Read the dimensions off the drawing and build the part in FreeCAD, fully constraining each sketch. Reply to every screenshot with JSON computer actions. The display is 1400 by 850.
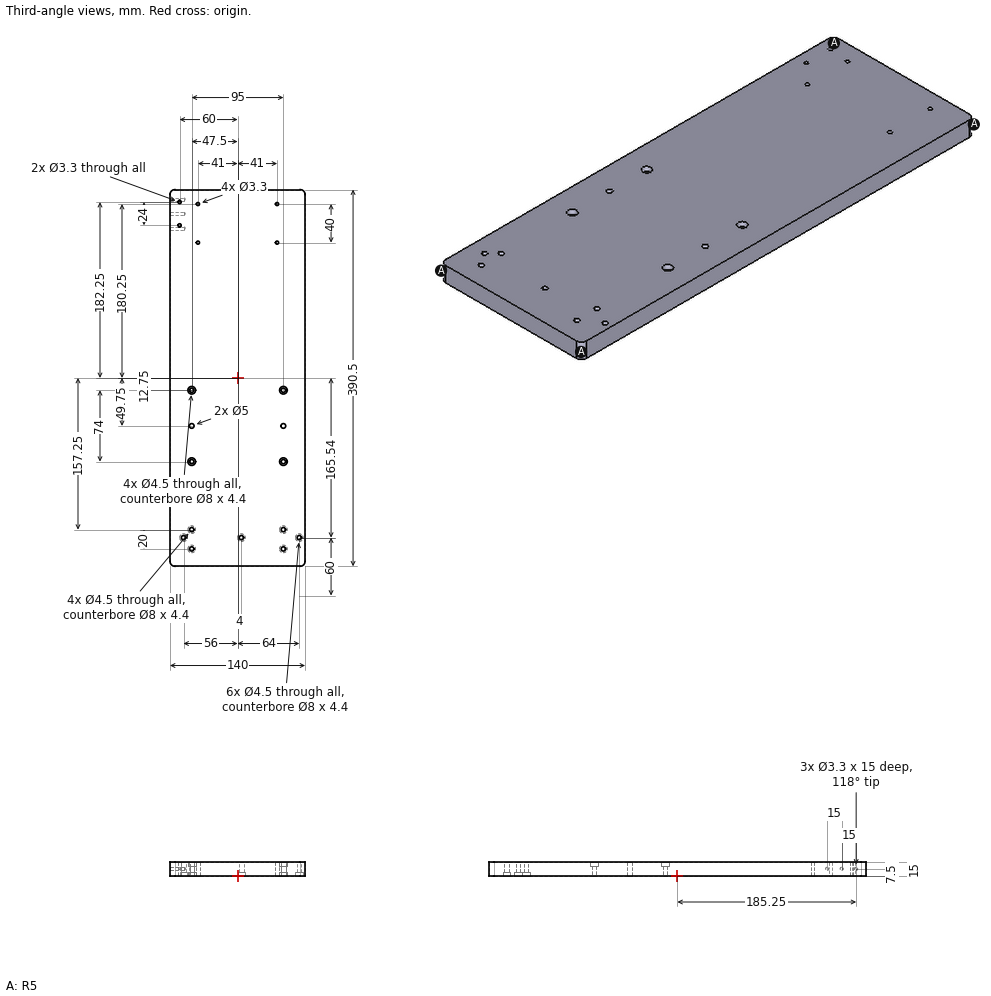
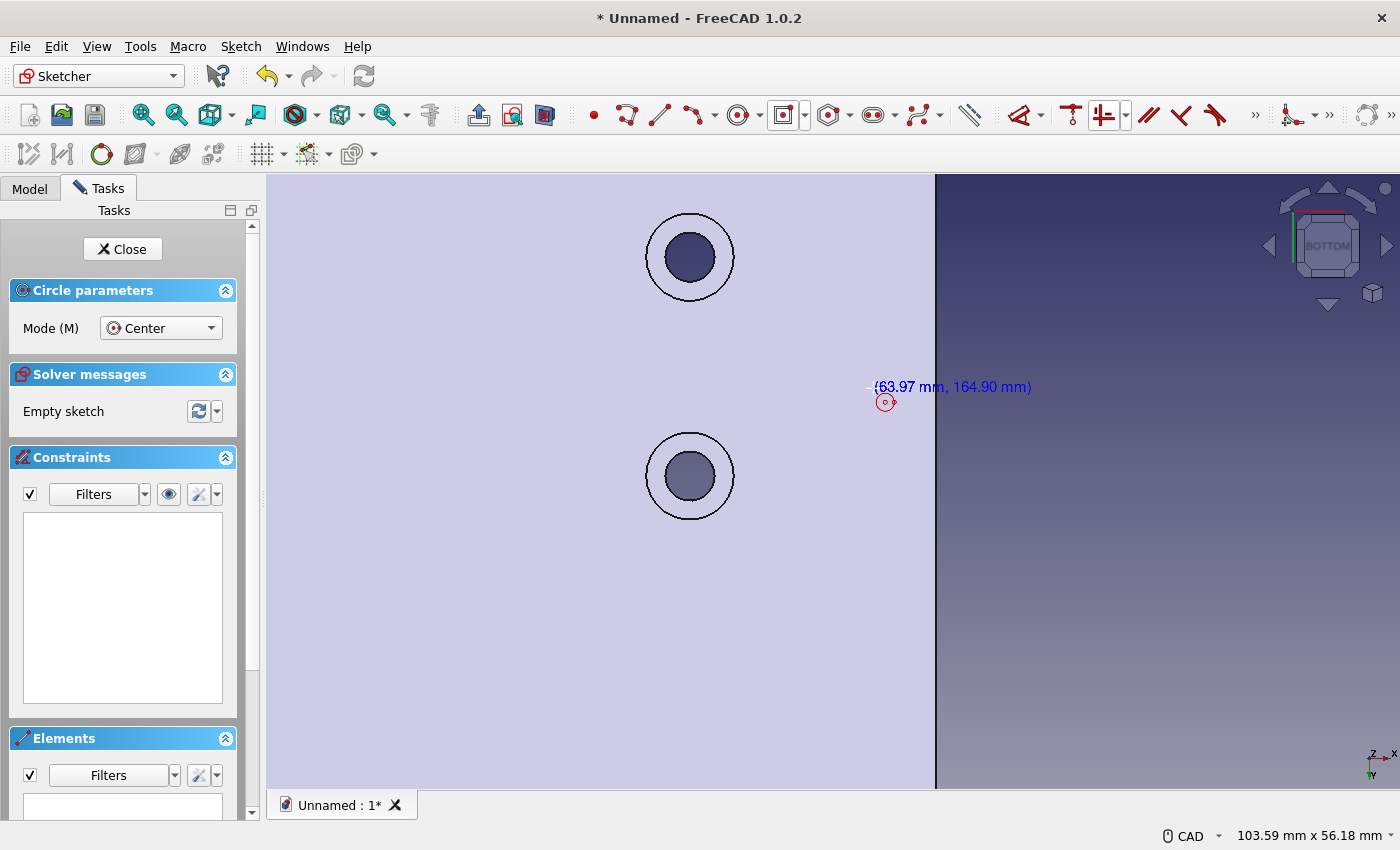
{"action": "scroll", "coordinate": [874, 389], "scroll_direction": "down", "scroll_amount": 9}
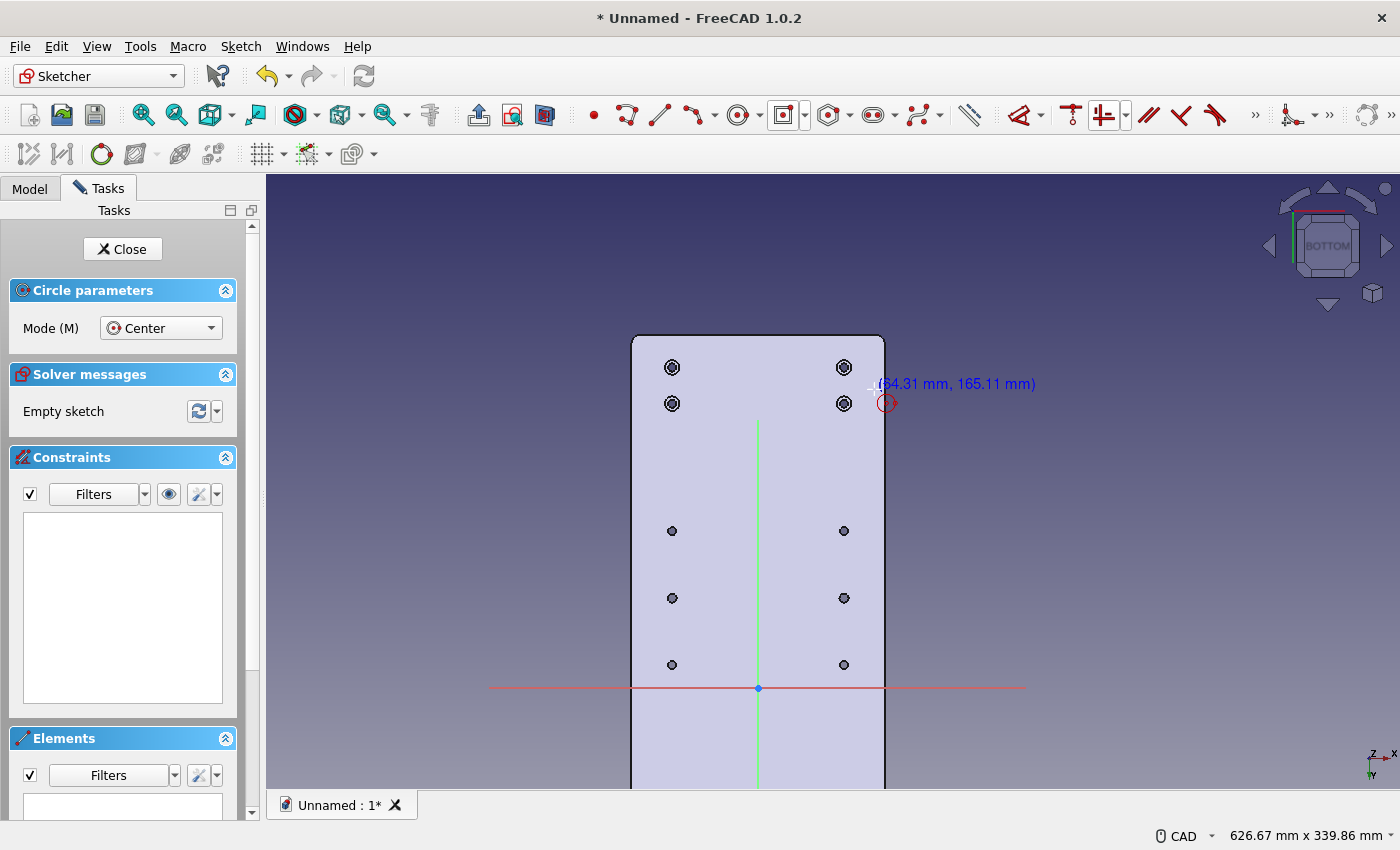
{"action": "left_click", "coordinate": [874, 389]}
{"action": "mouse_move", "coordinate": [877, 386]}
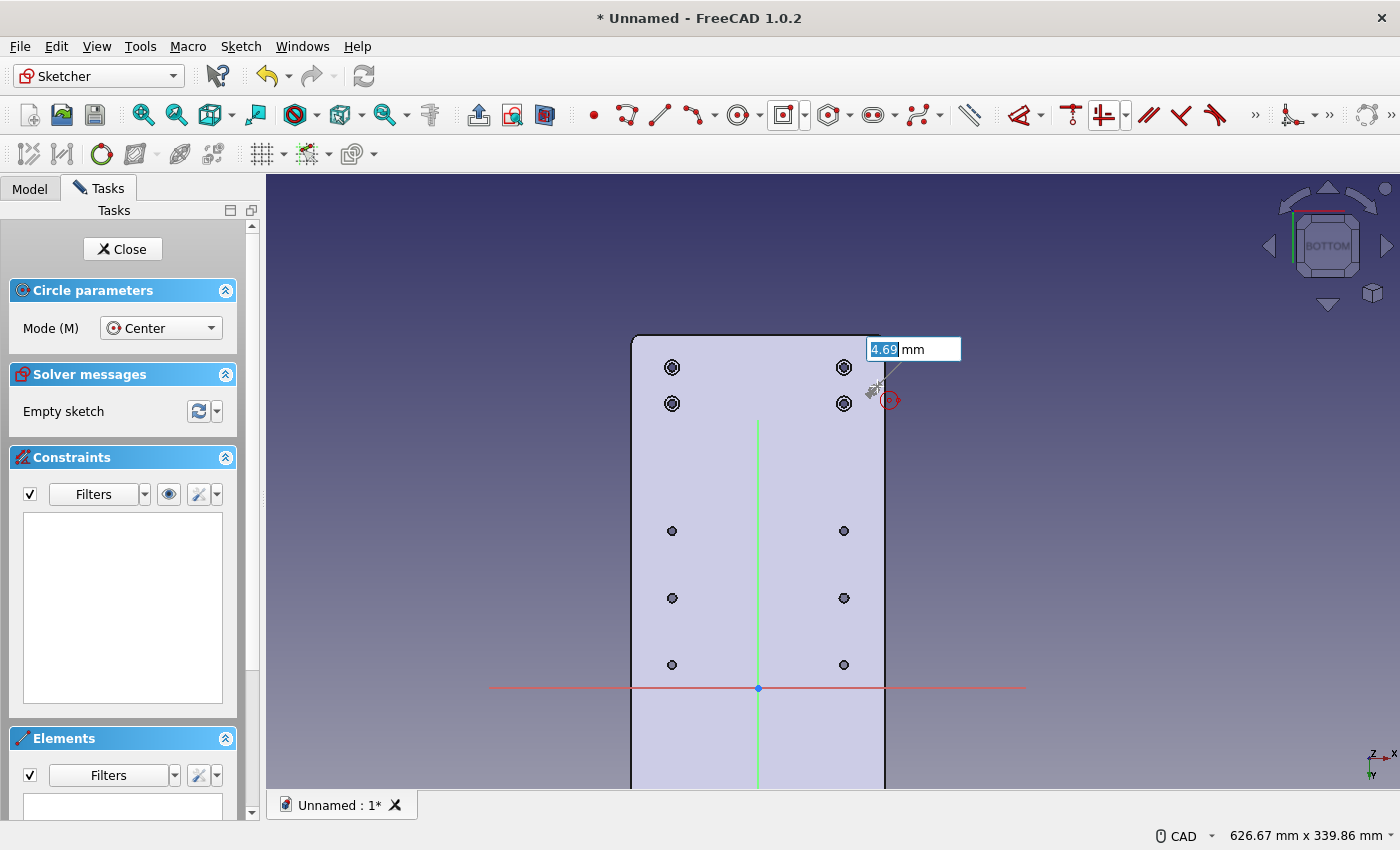
{"action": "type", "text": "4.5"}
{"action": "key", "text": "Return"}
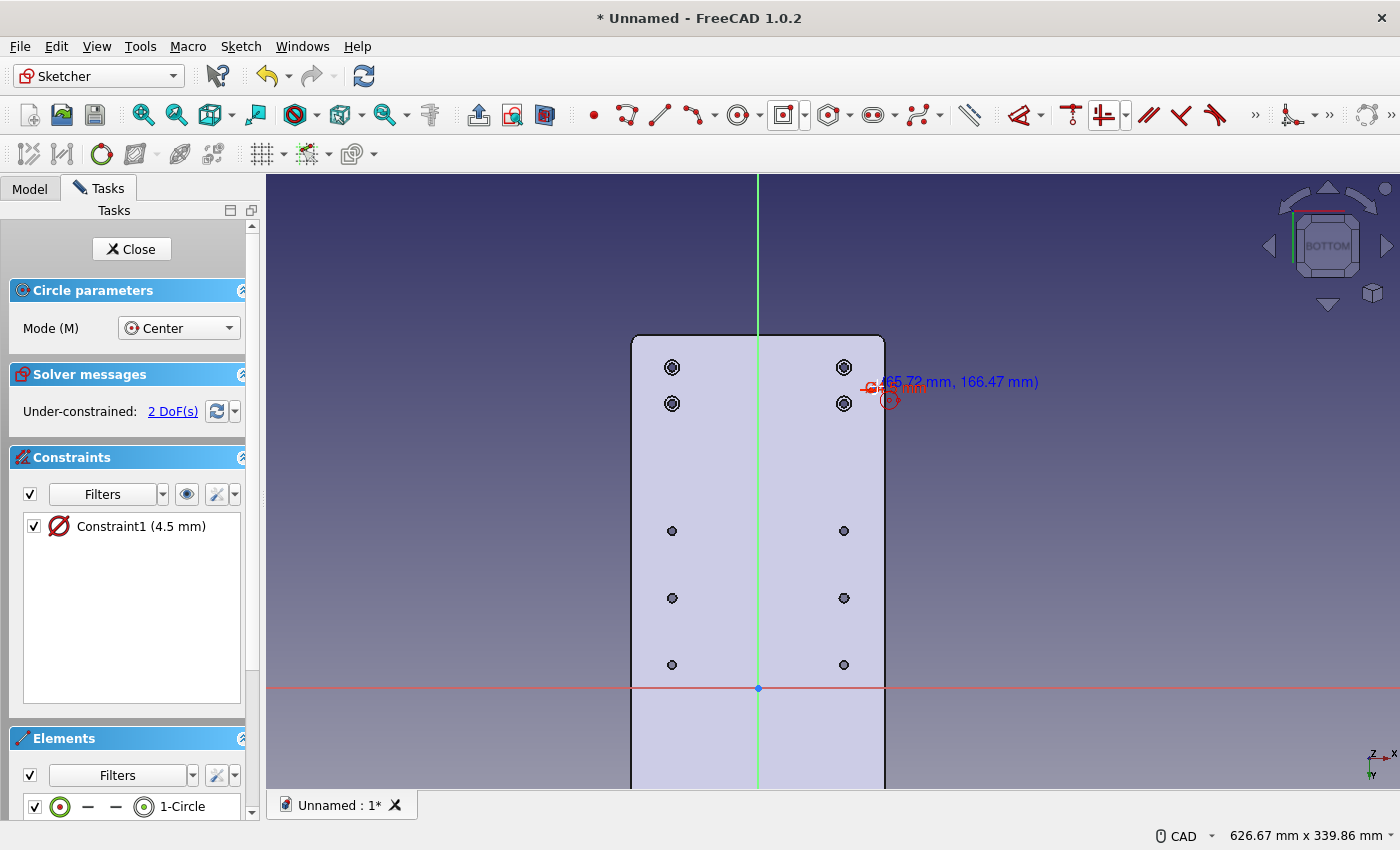
{"action": "scroll", "coordinate": [765, 389], "scroll_direction": "up", "scroll_amount": 9}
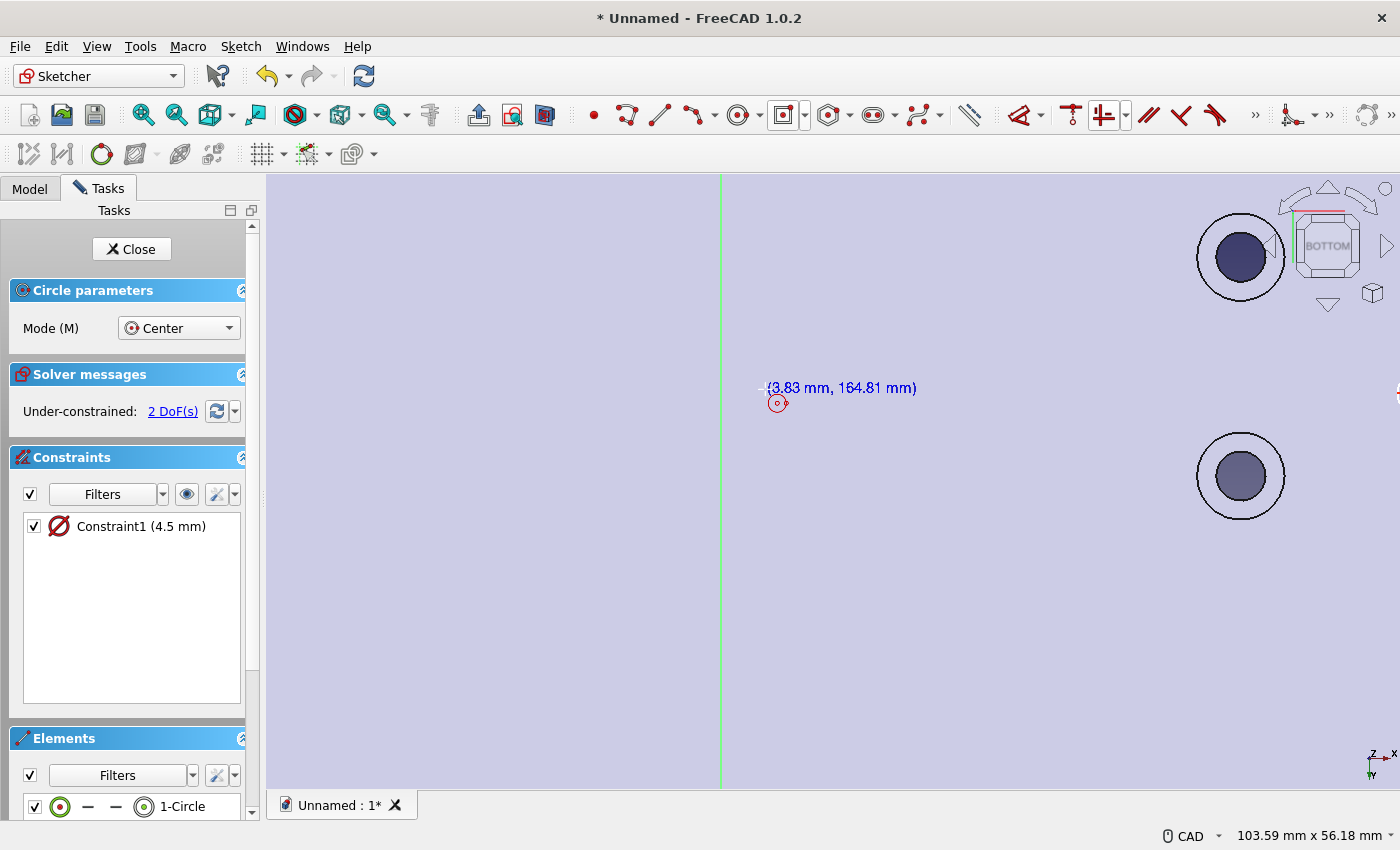
{"action": "left_click", "coordinate": [765, 385]}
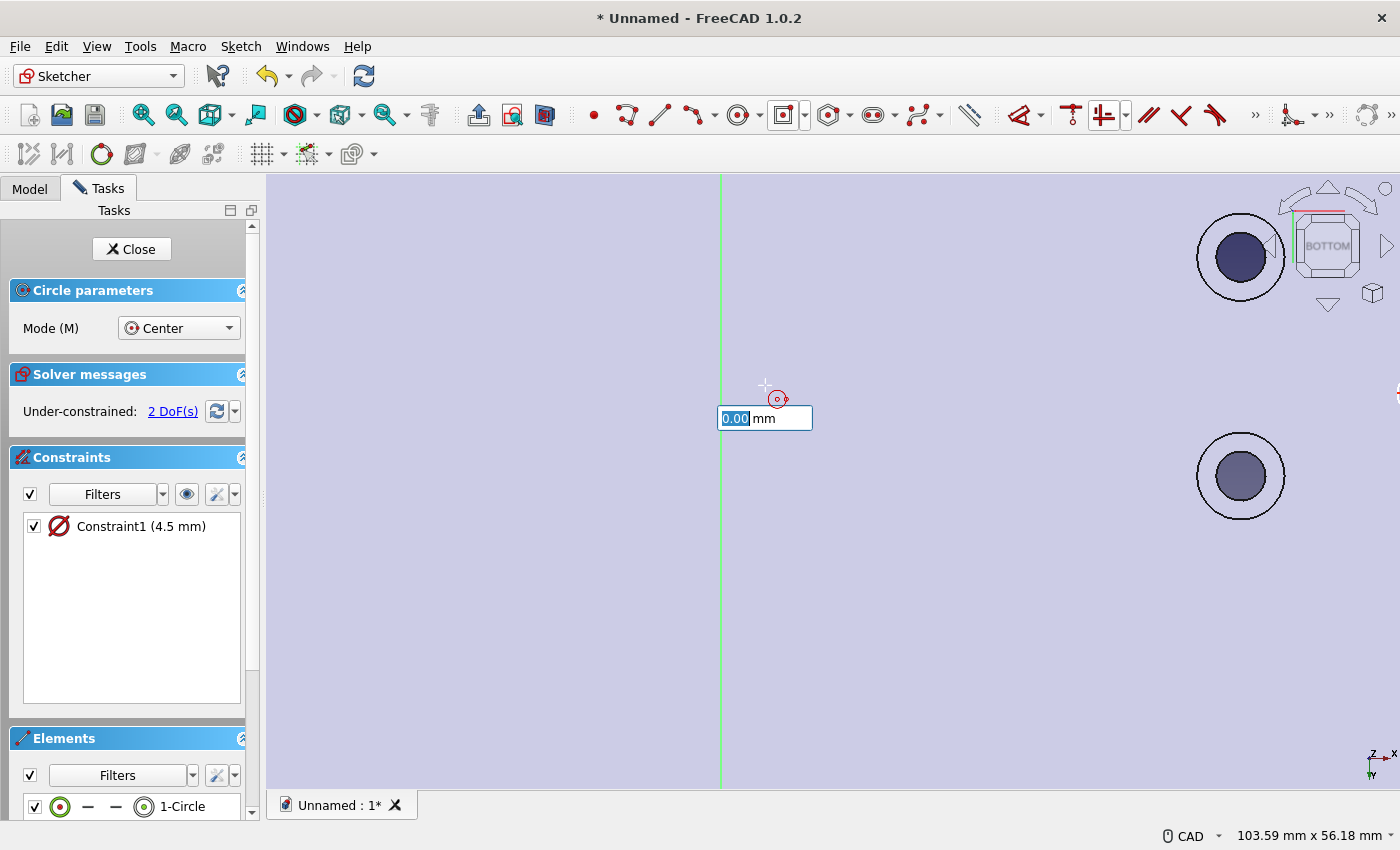
{"action": "scroll", "coordinate": [764, 389], "scroll_direction": "down", "scroll_amount": 9}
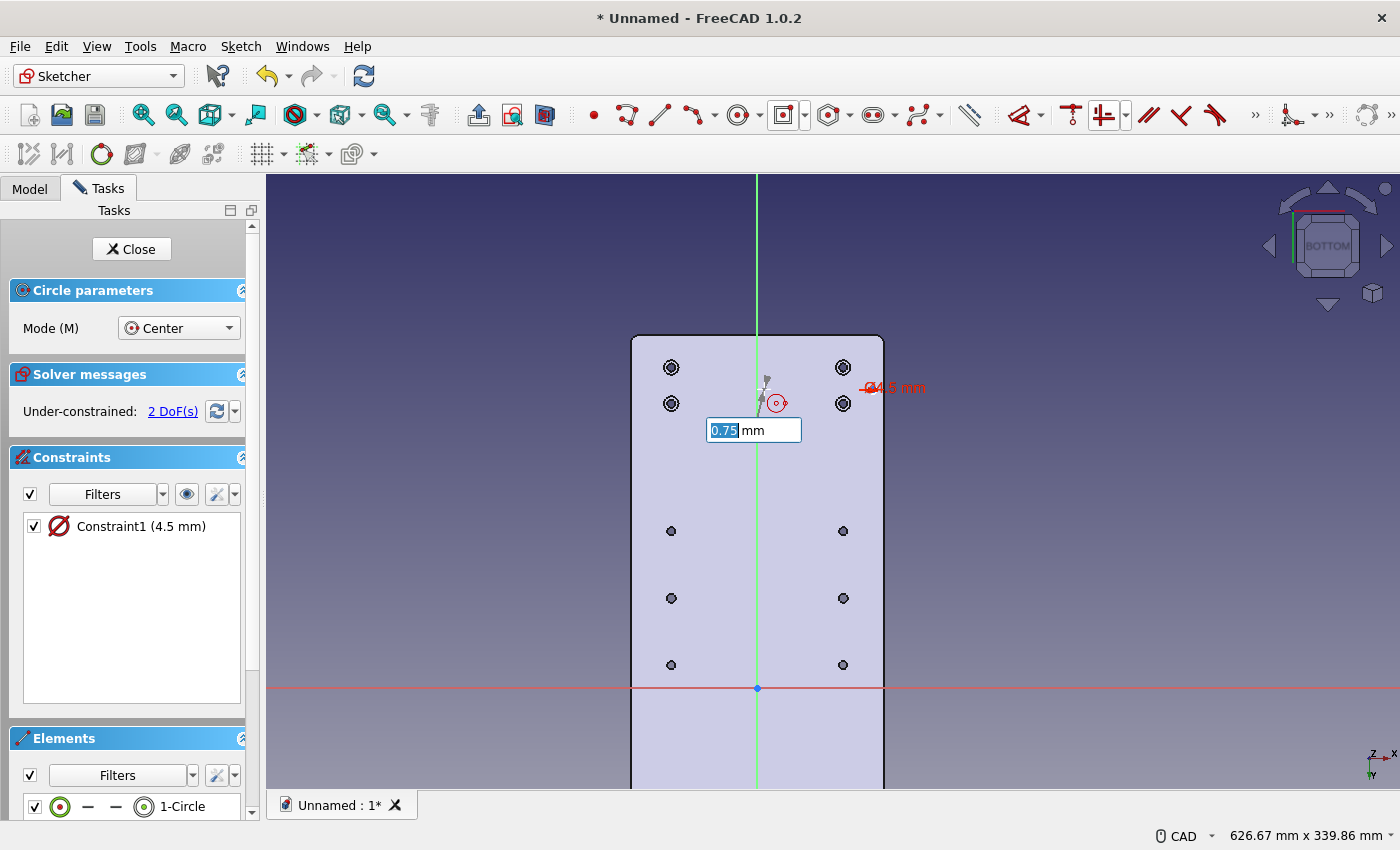
{"action": "scroll", "coordinate": [767, 386], "scroll_direction": "up", "scroll_amount": 3}
{"action": "mouse_move", "coordinate": [767, 385]}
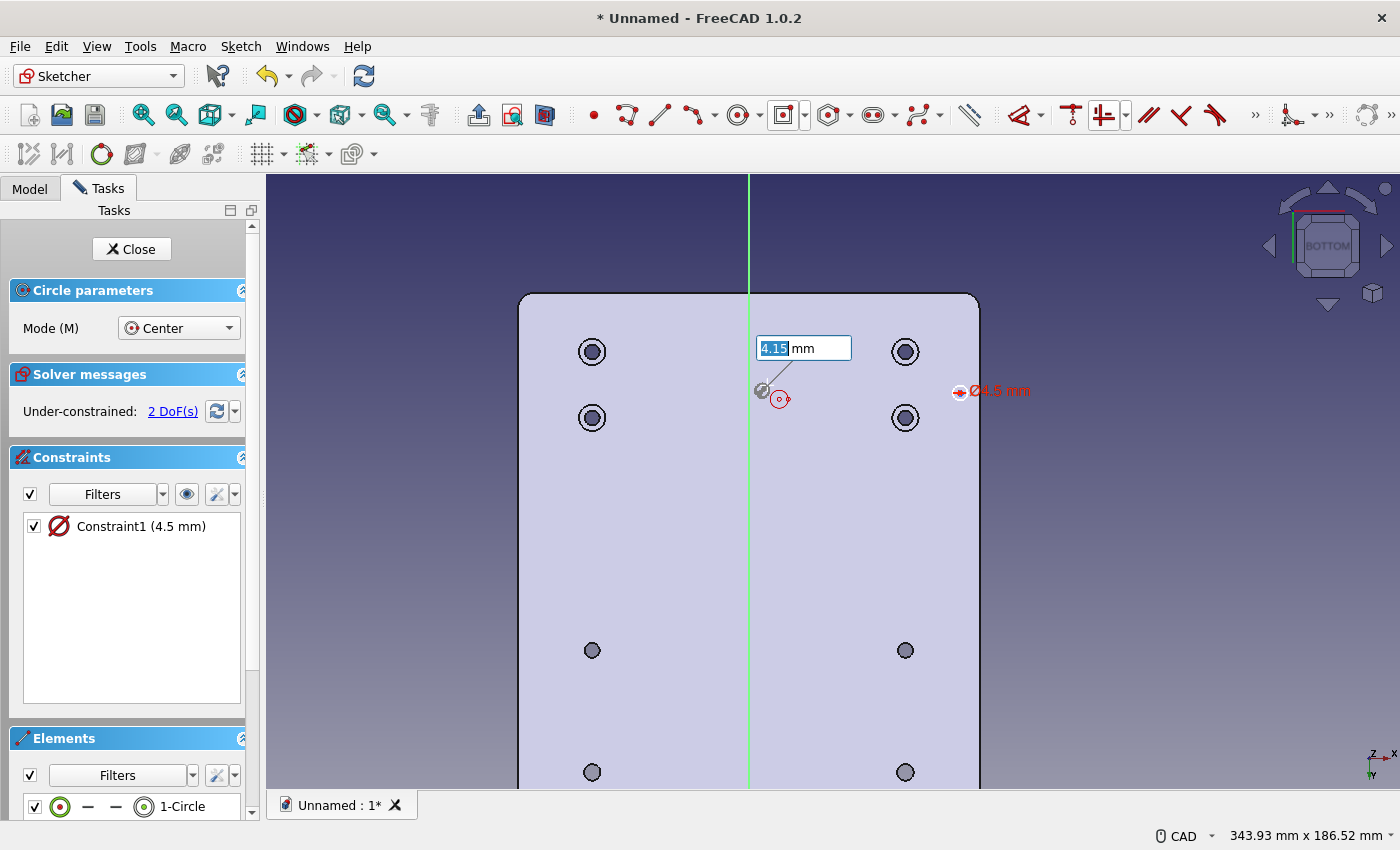
{"action": "type", "text": "4.5"}
{"action": "key", "text": "Return"}